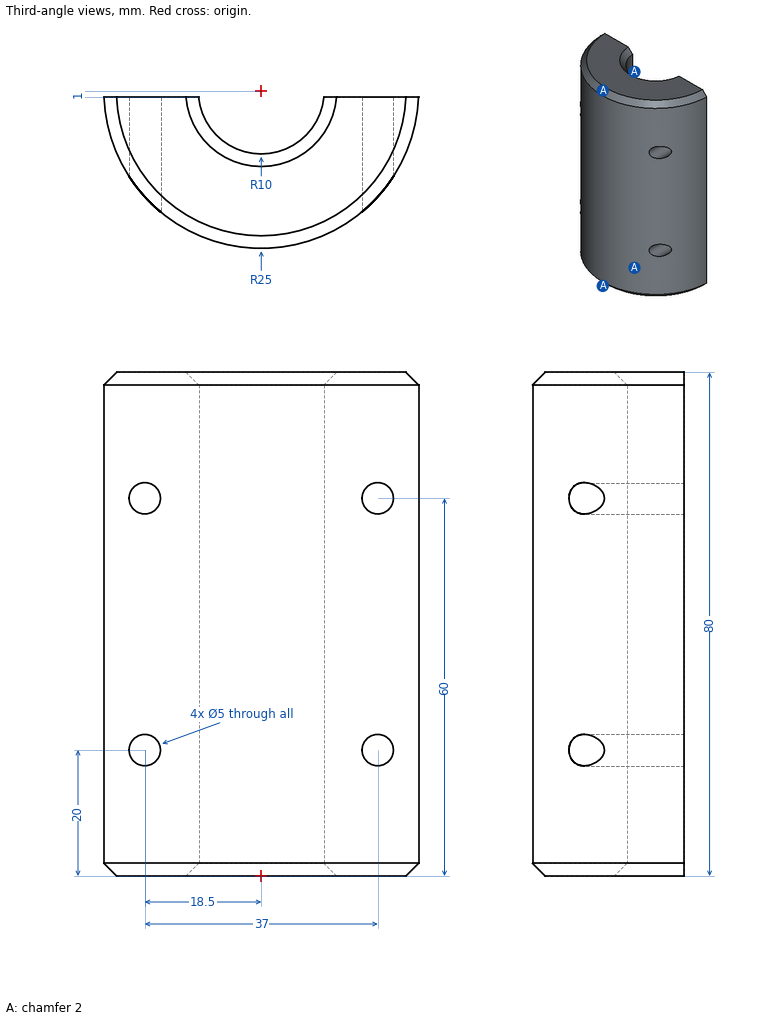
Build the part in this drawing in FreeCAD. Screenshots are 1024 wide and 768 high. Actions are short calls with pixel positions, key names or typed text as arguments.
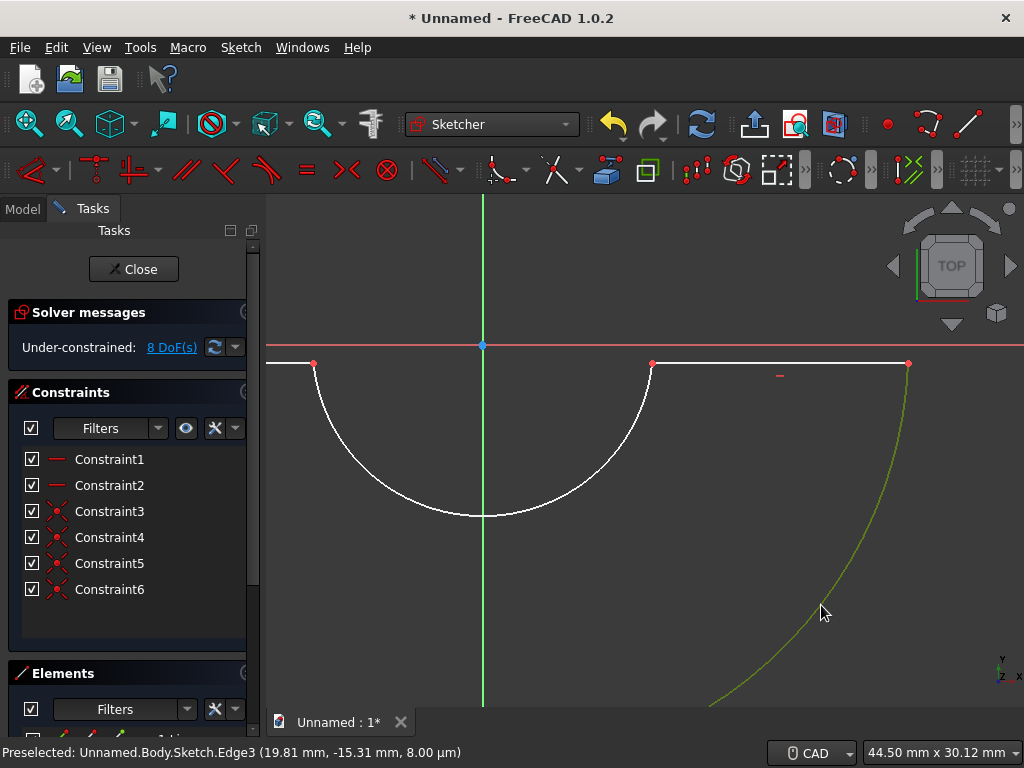
click(388, 488)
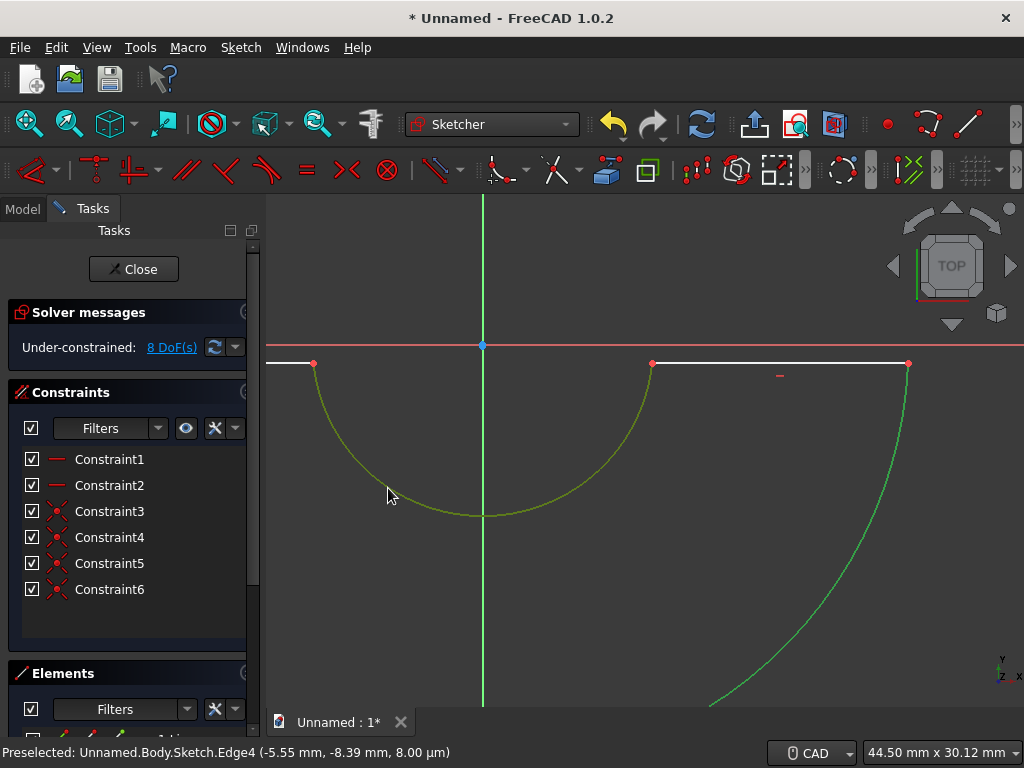
click(94, 170)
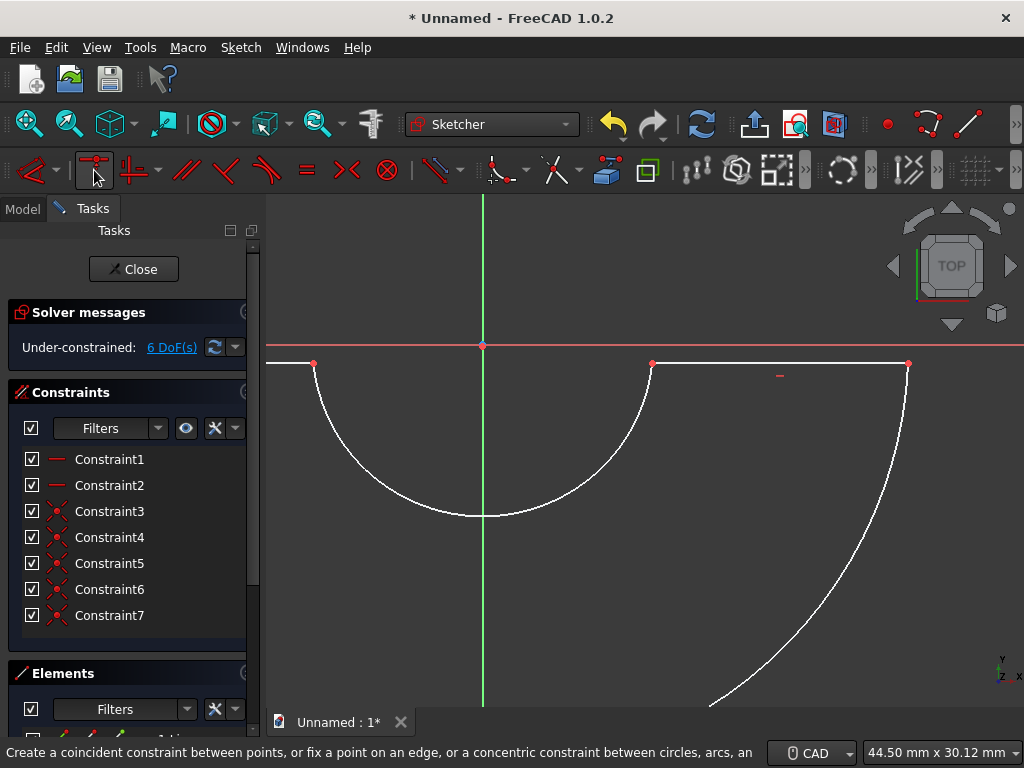
drag(473, 335, 493, 356)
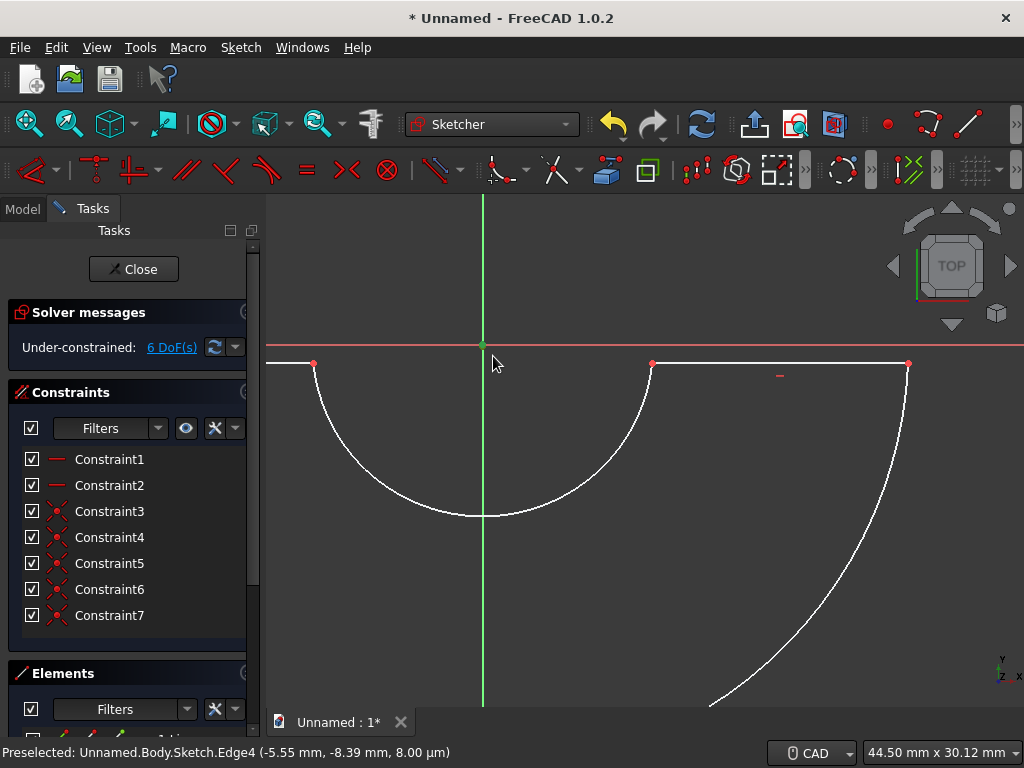
click(94, 170)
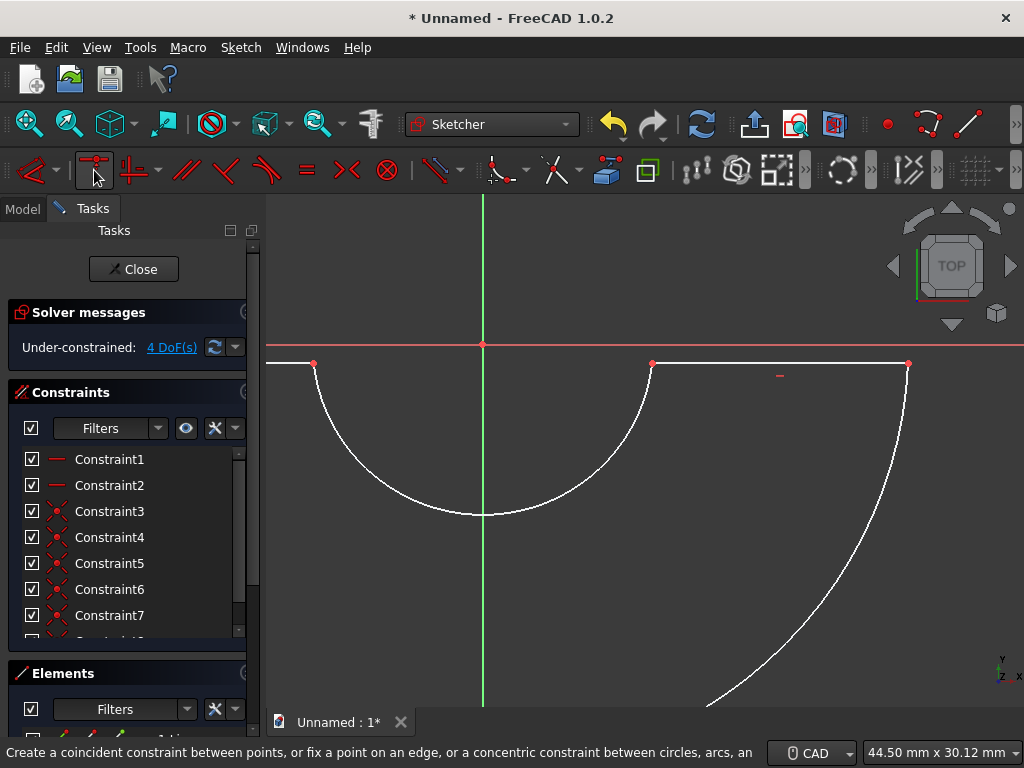
click(32, 170)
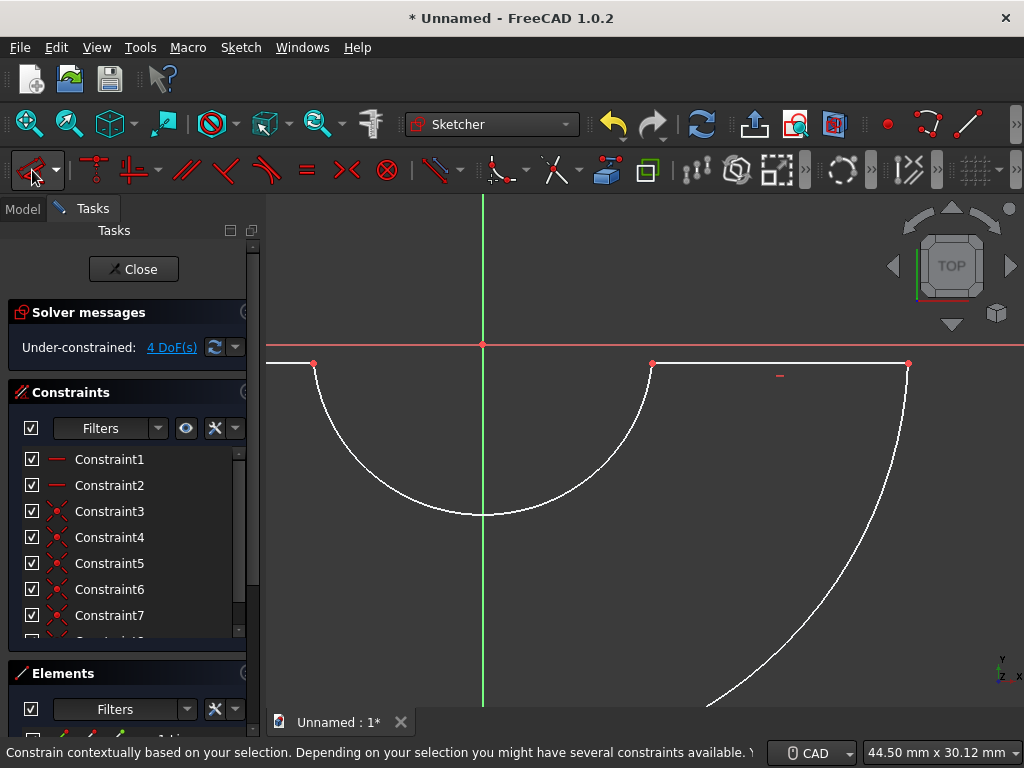
click(821, 604)
click(846, 623)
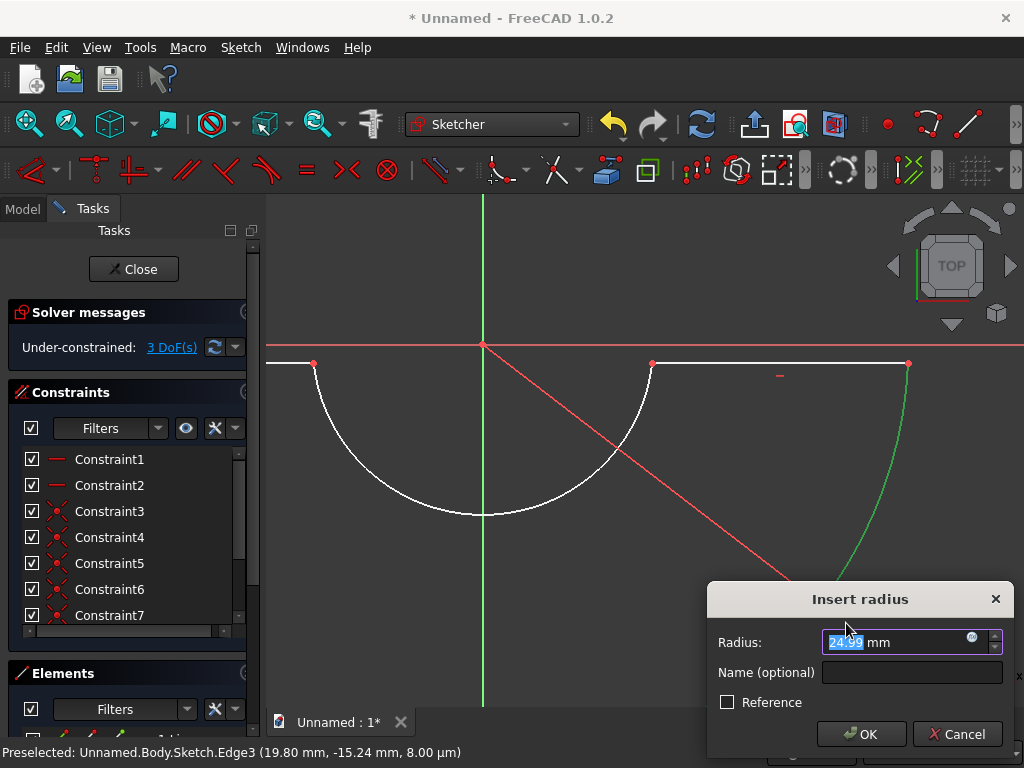
text(25)
key(Return)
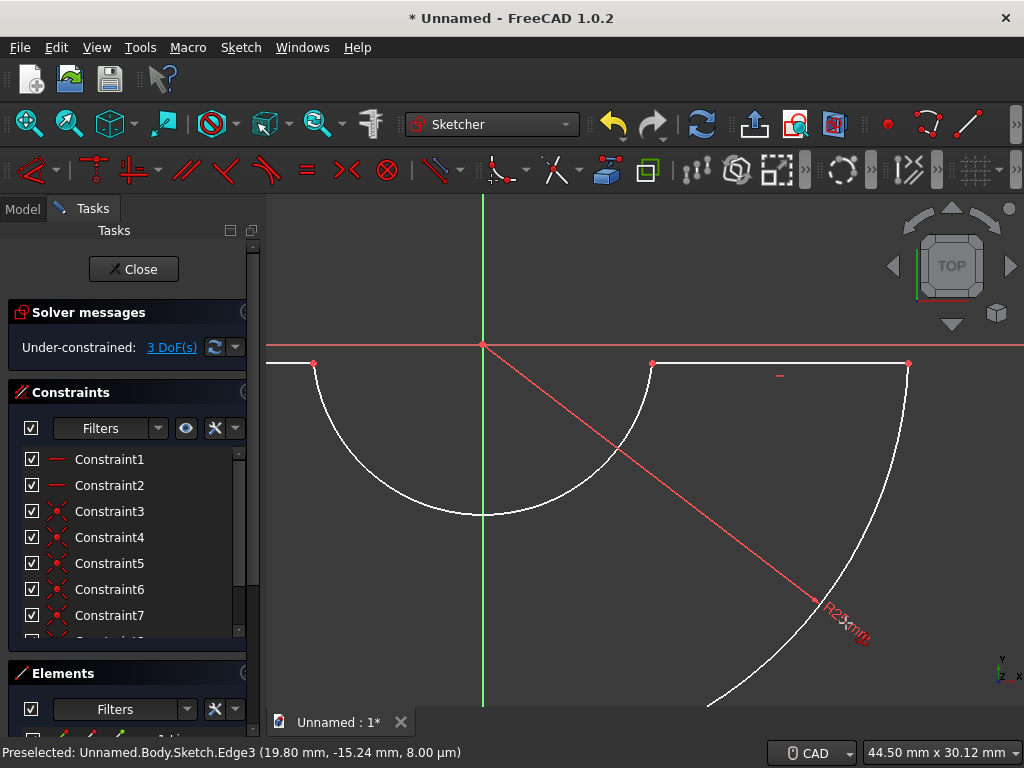
click(389, 487)
click(371, 514)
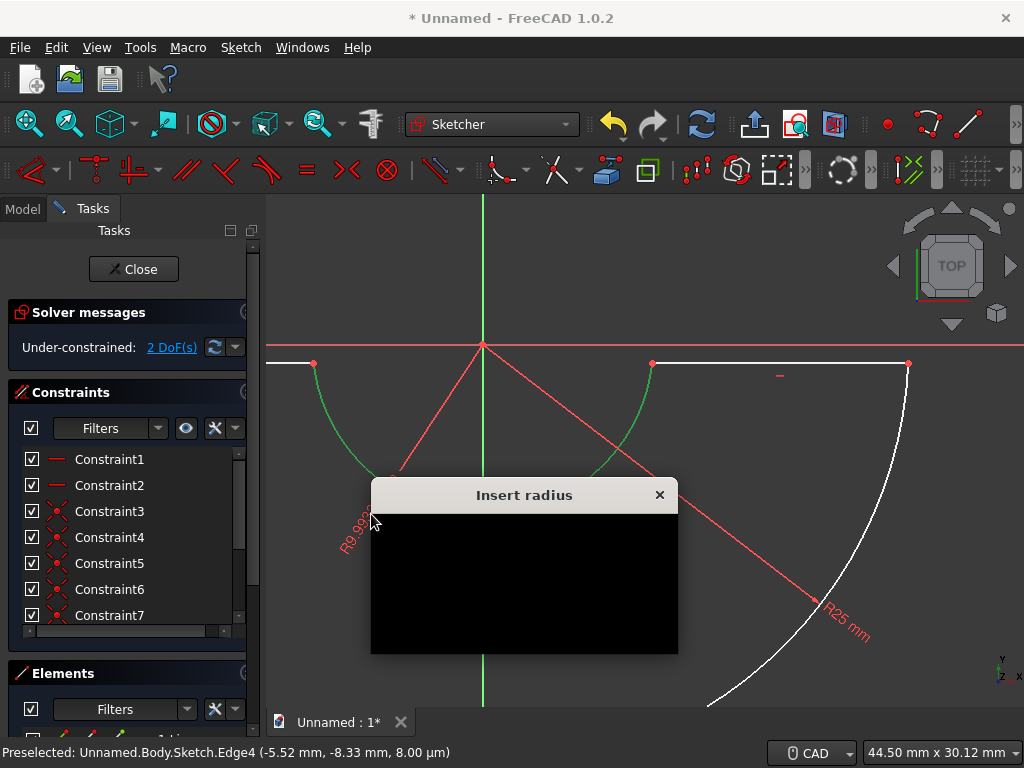
text(10)
key(Return)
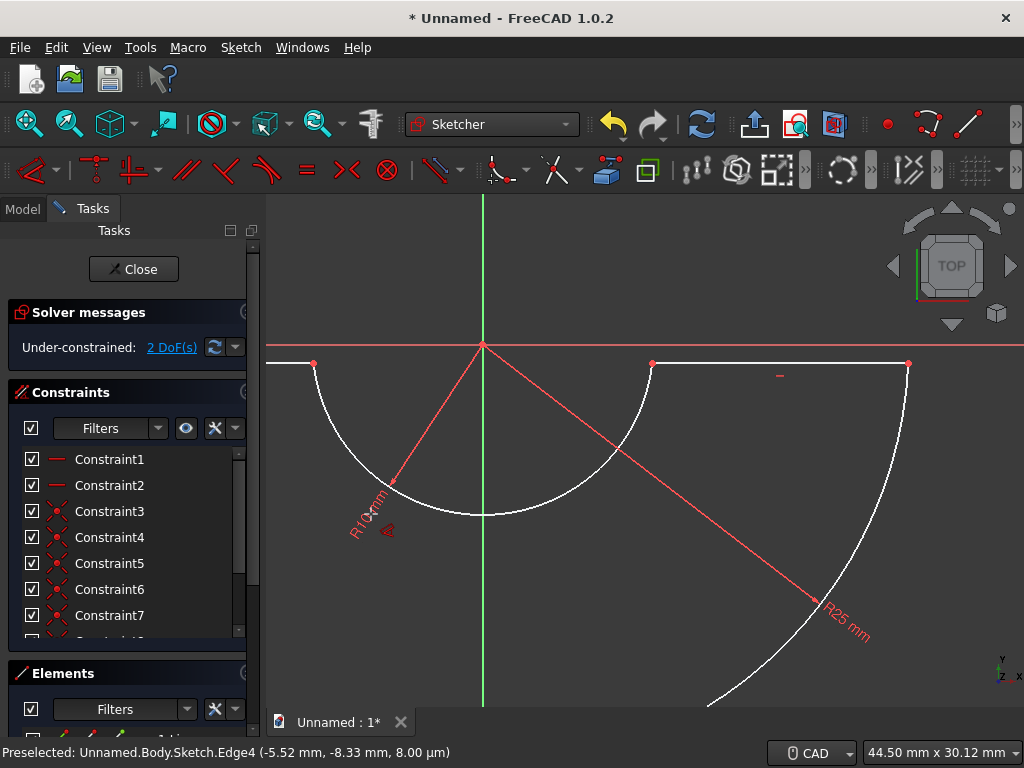
scroll(314, 363, up, 5)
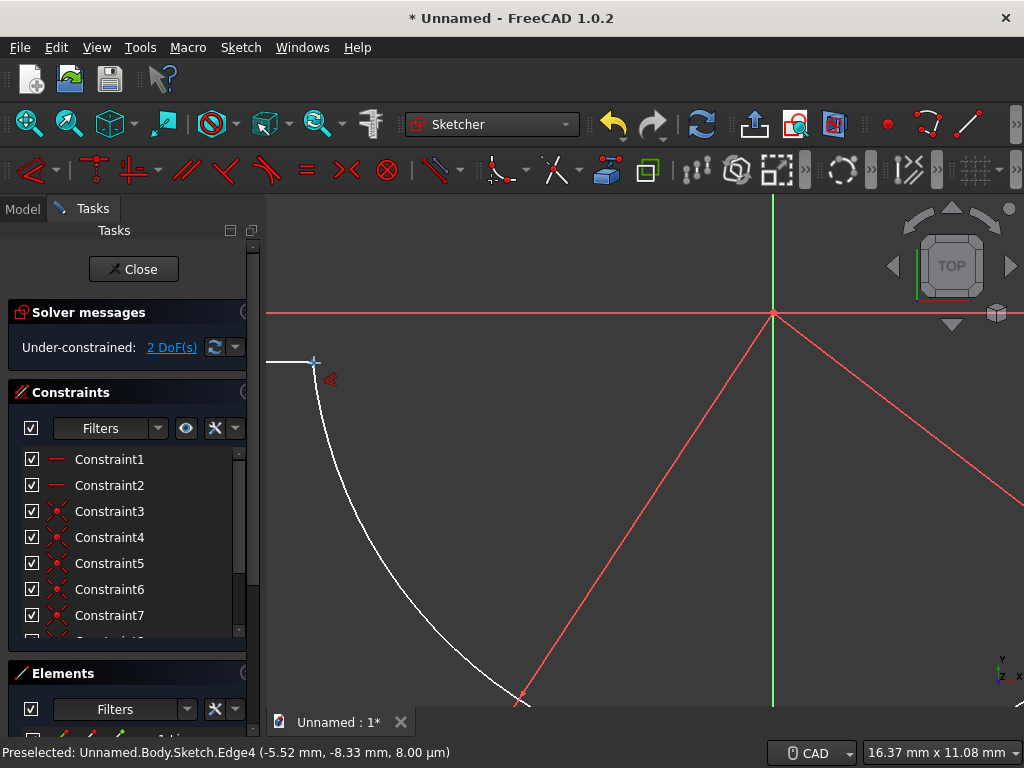
click(313, 362)
click(807, 338)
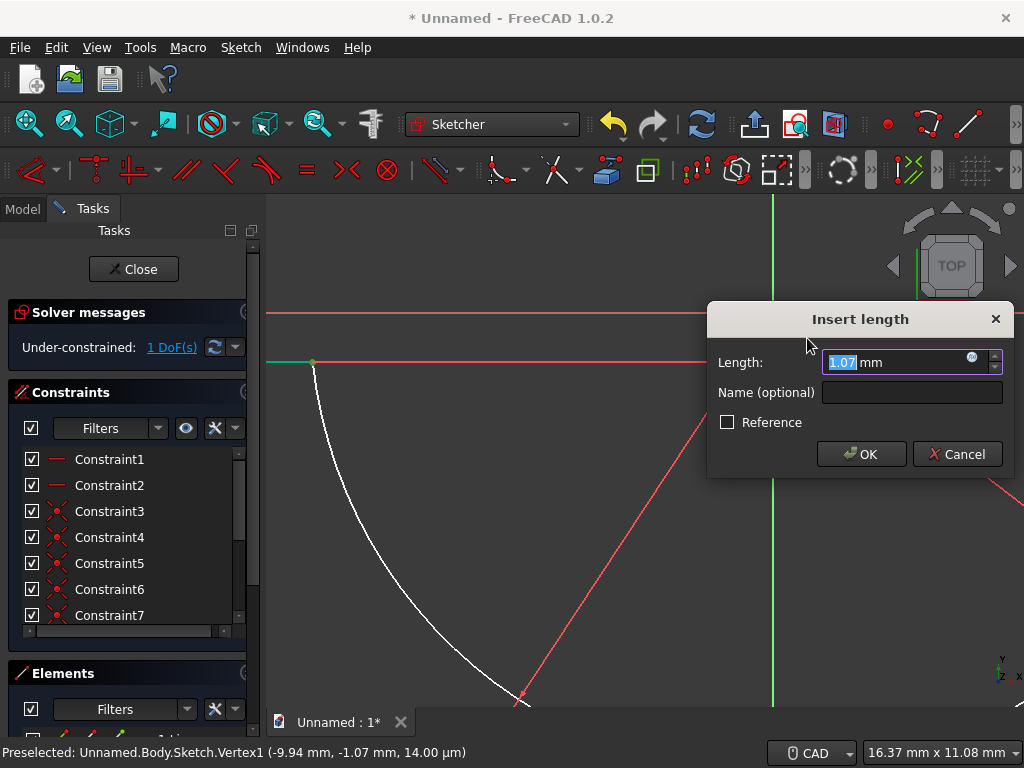
text(1)
key(Return)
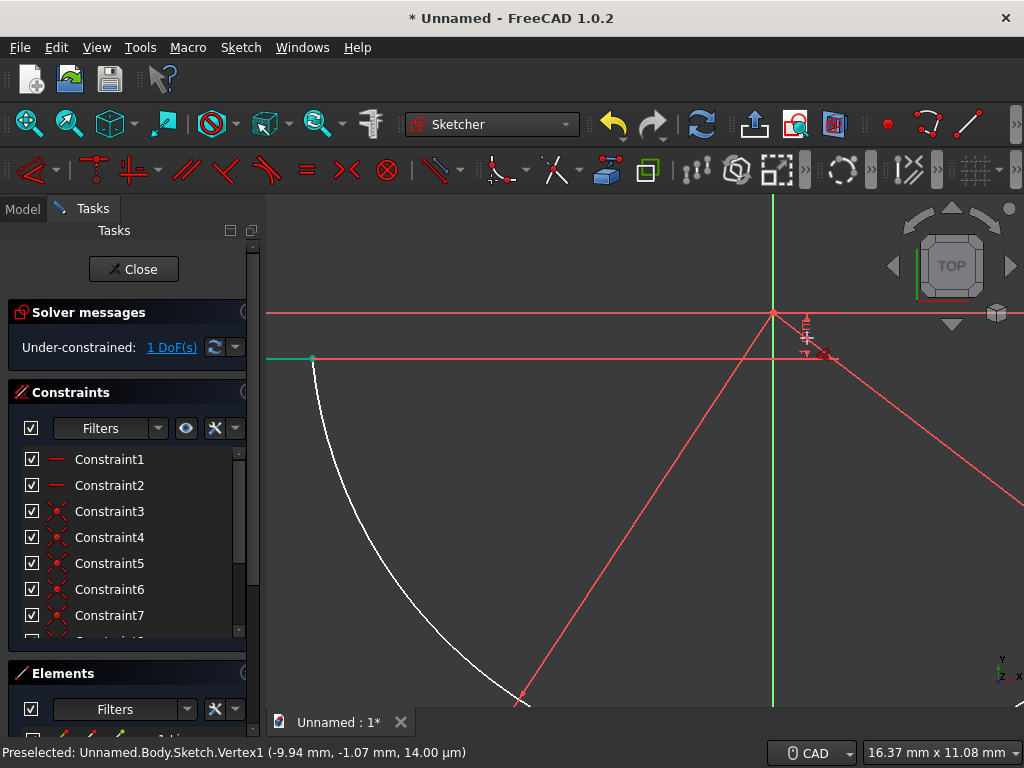
scroll(538, 363, down, 9)